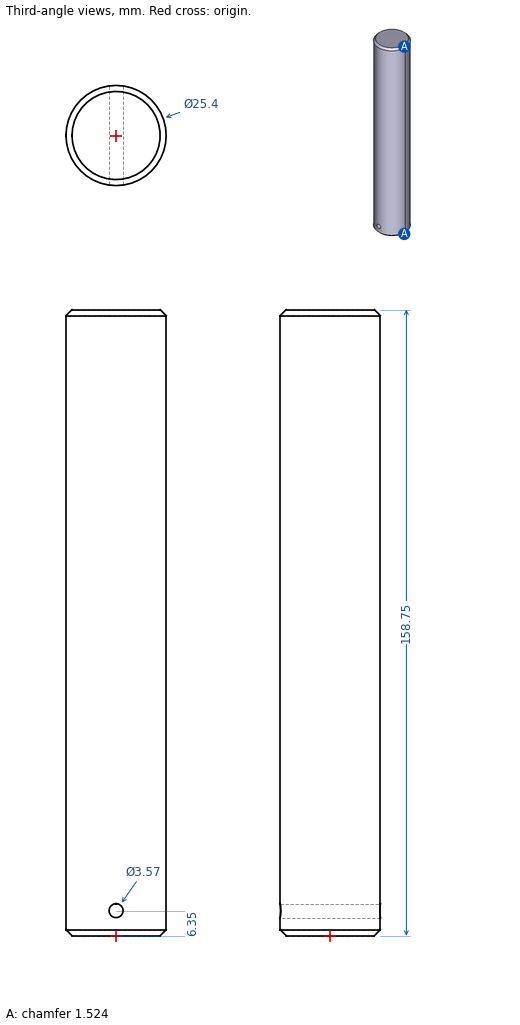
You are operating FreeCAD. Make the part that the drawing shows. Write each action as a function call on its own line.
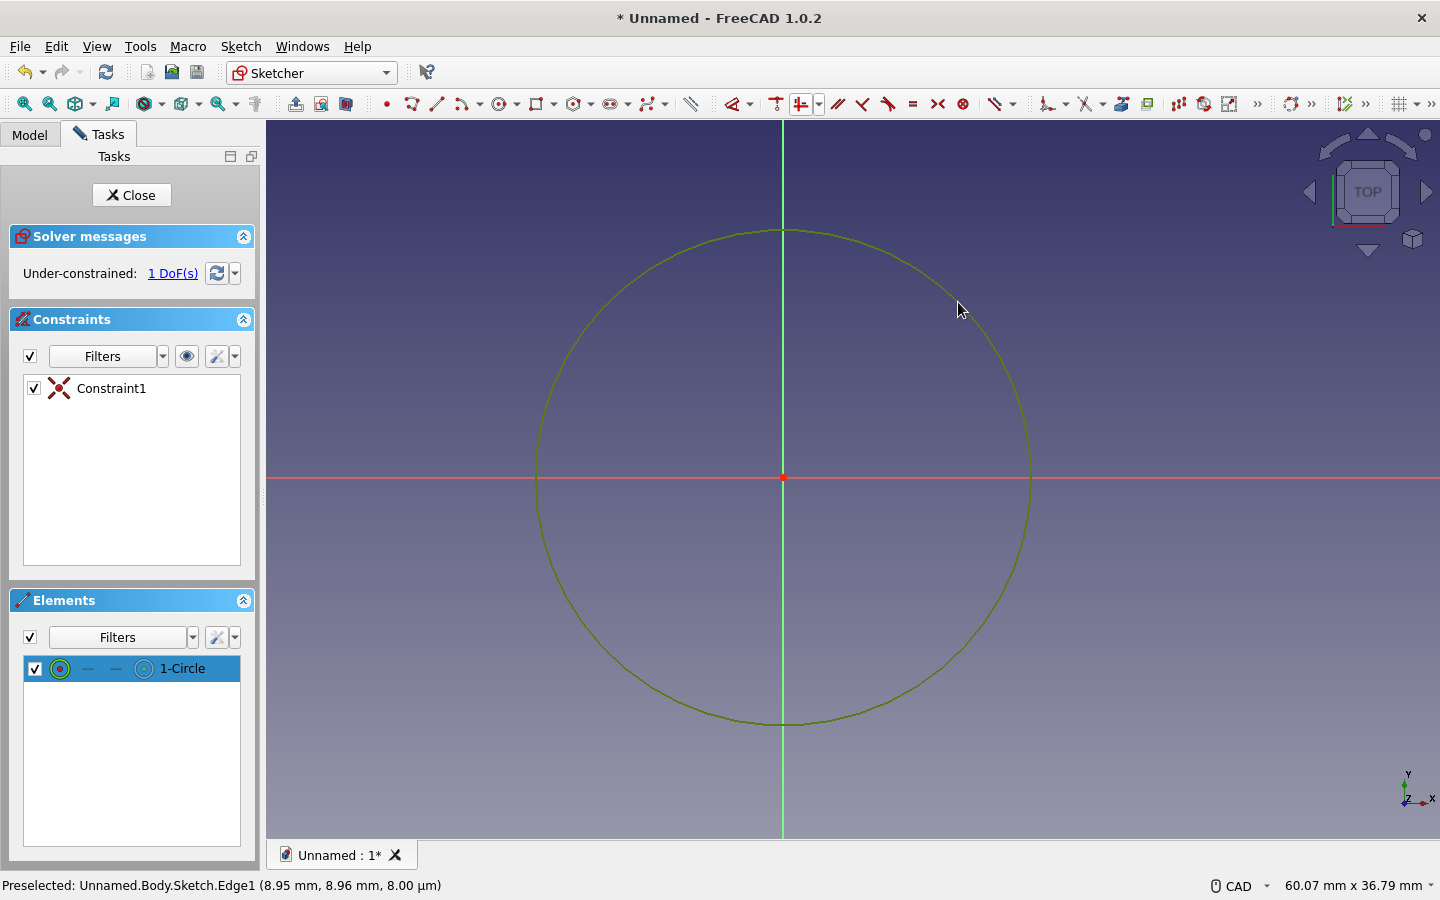
key(k)
key(o)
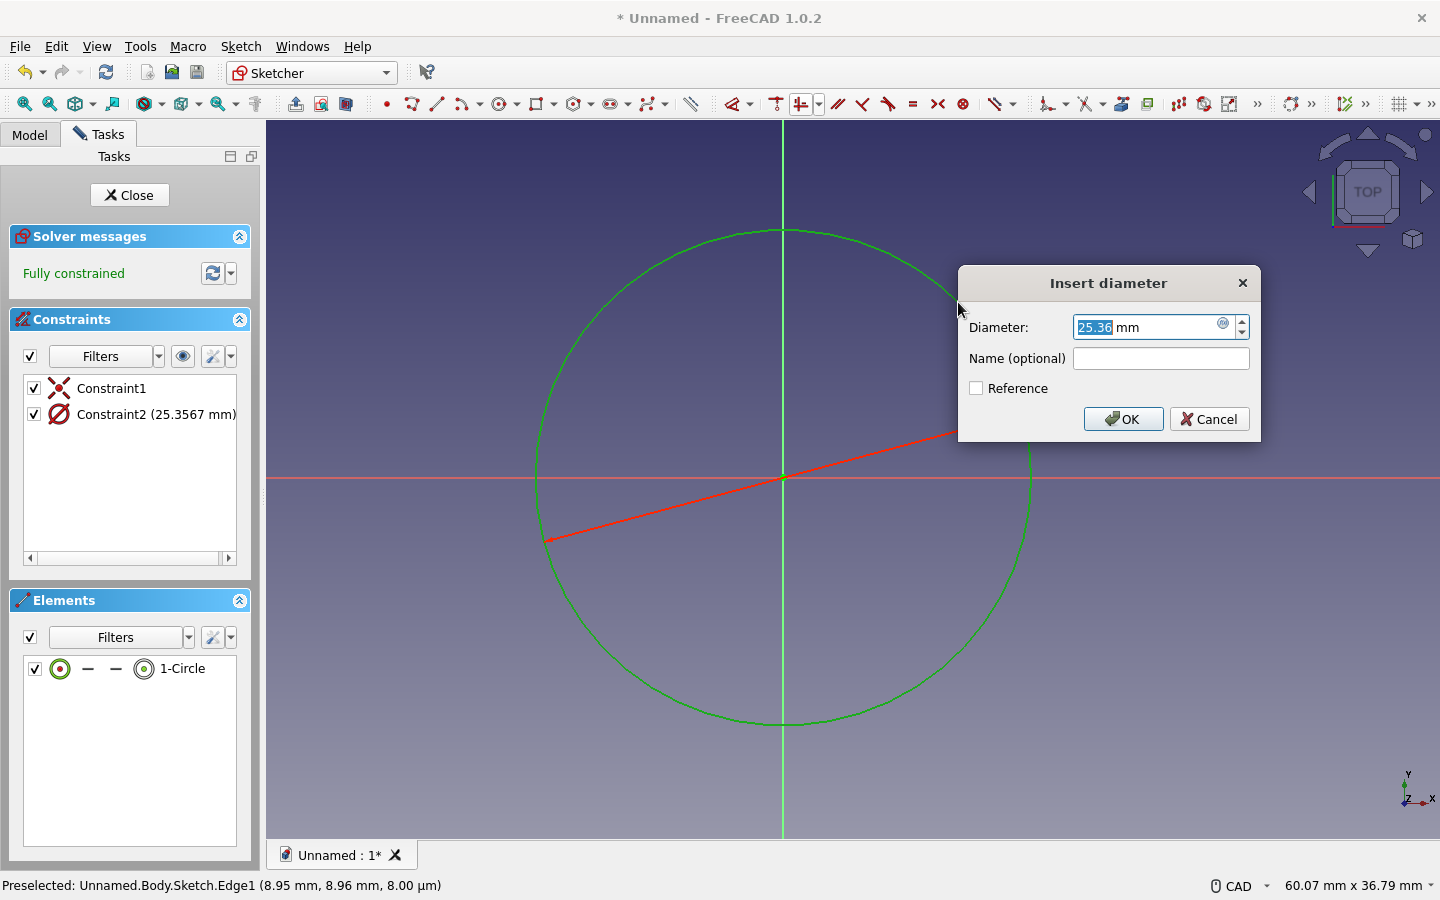
text(25.4)
key(Return)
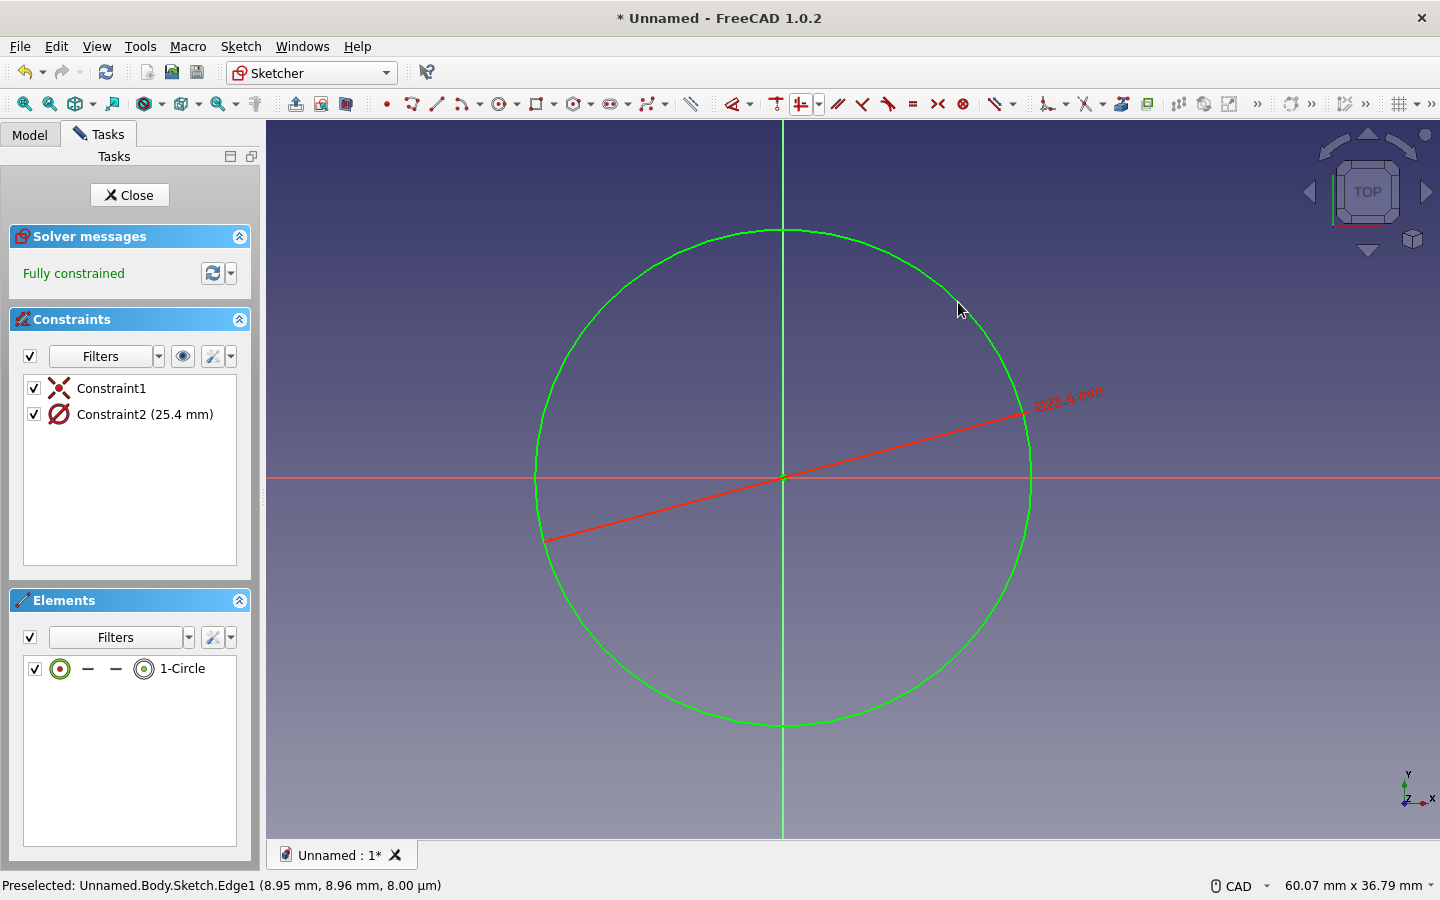
click(130, 195)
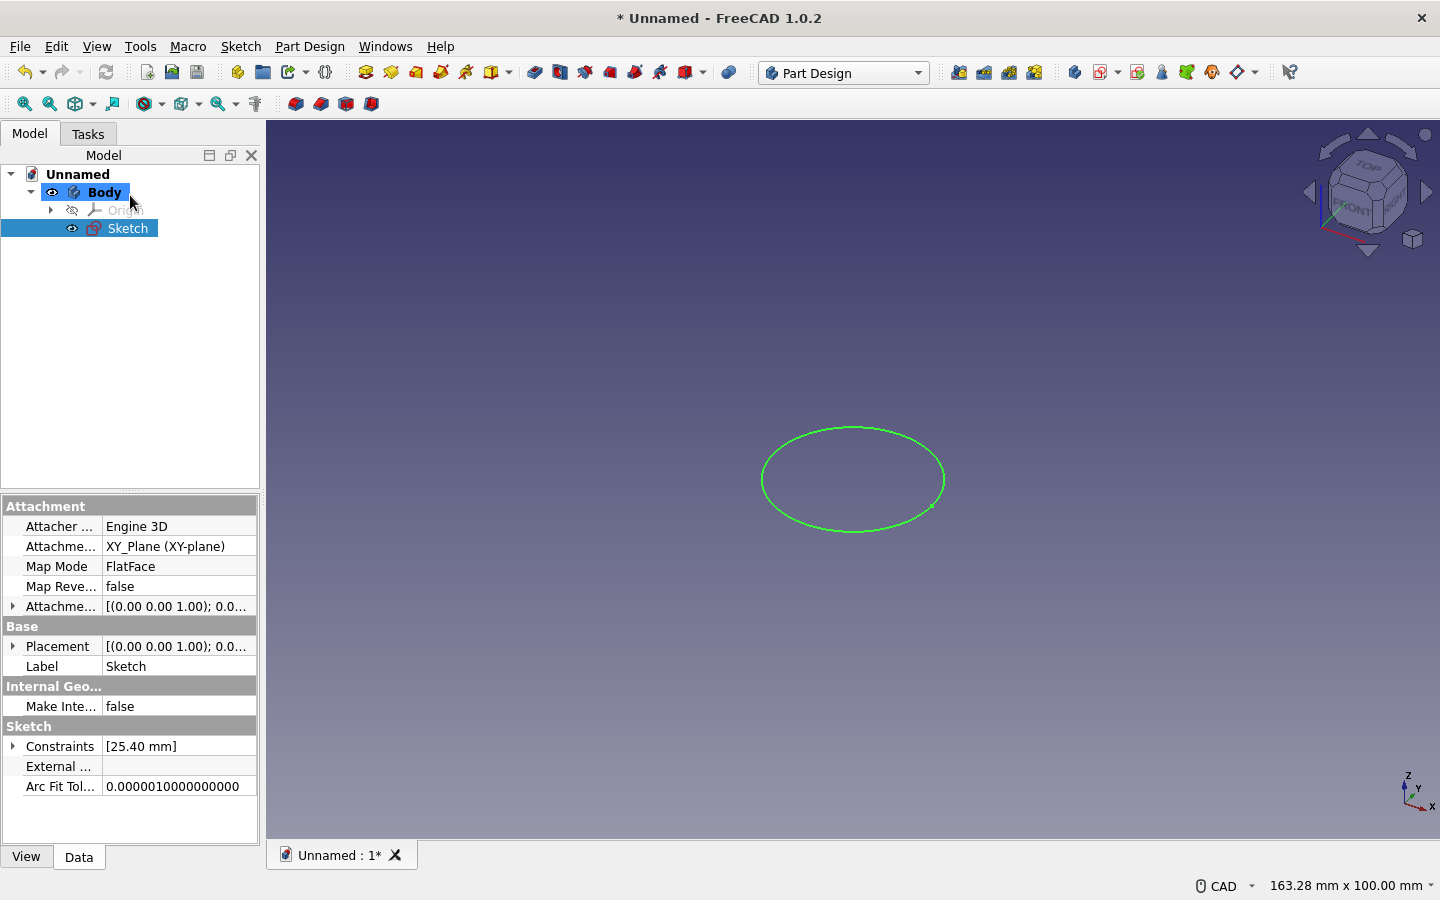
click(366, 72)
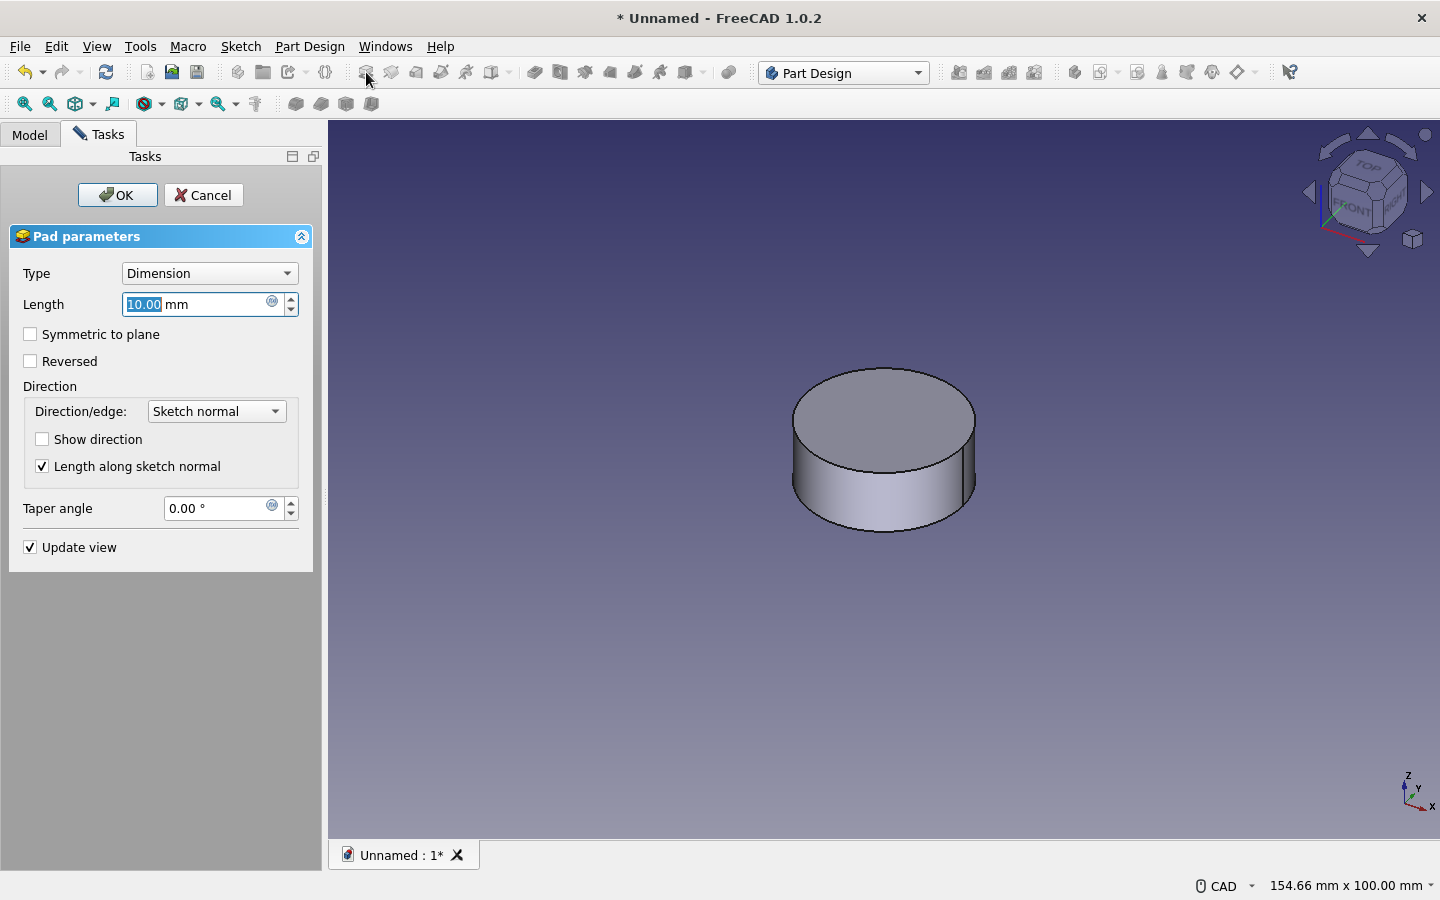
text(158.75)
key(Tab)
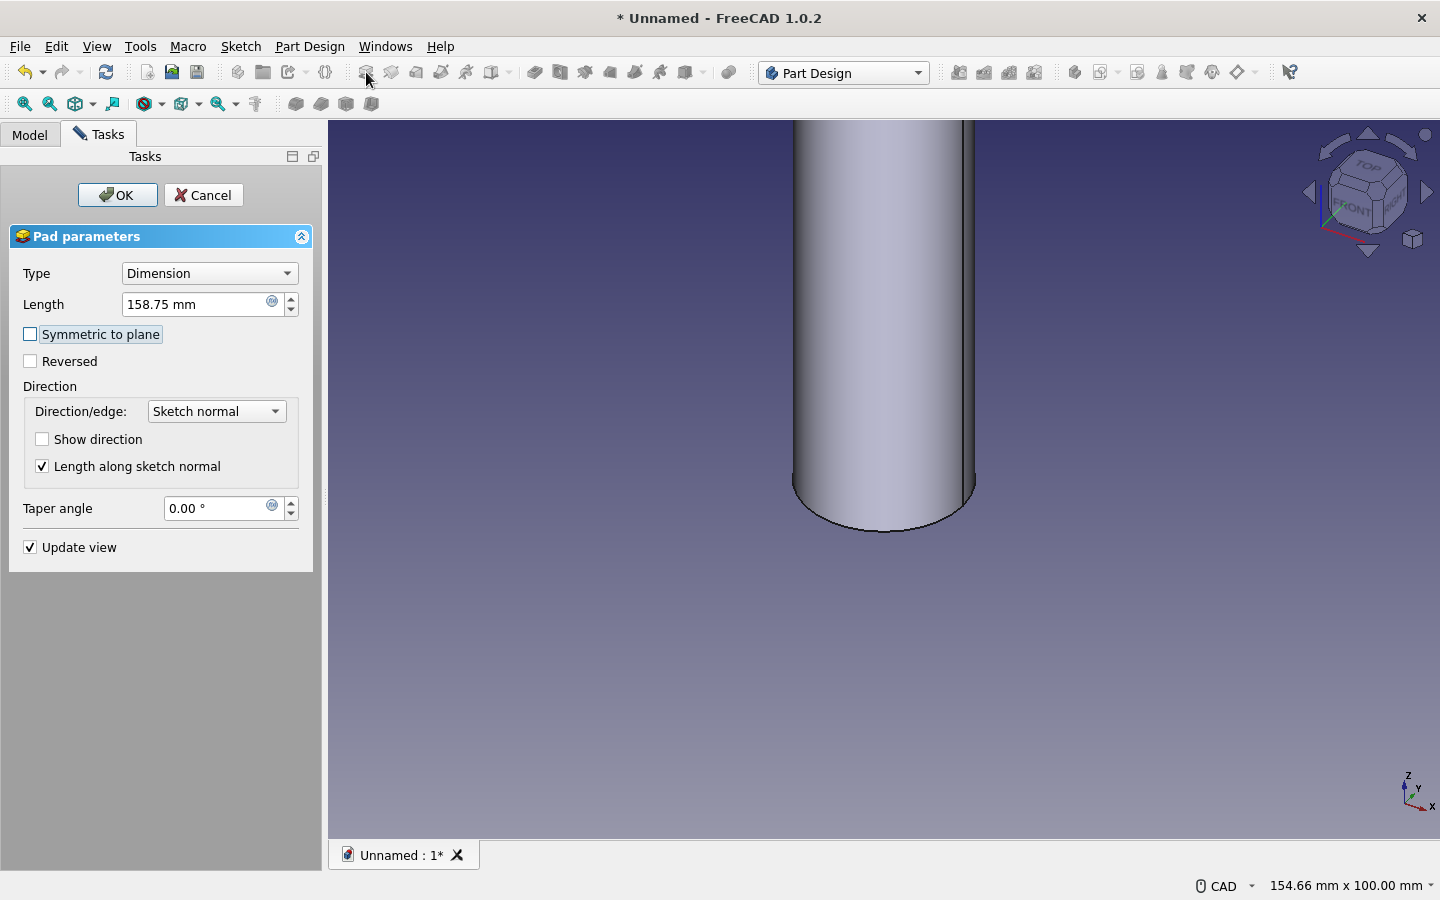
click(118, 195)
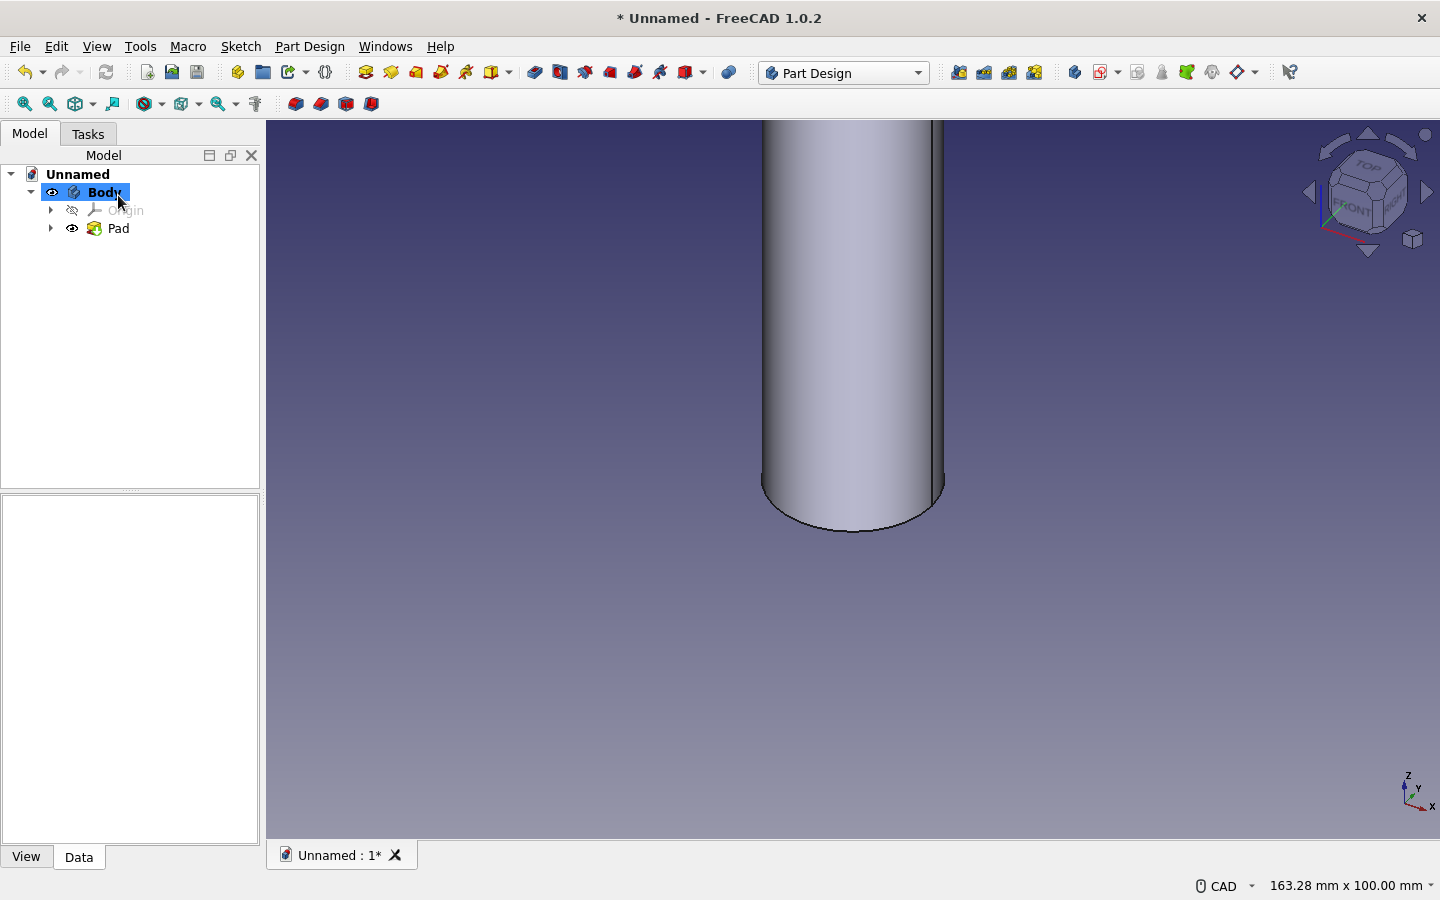
key(v)
key(f)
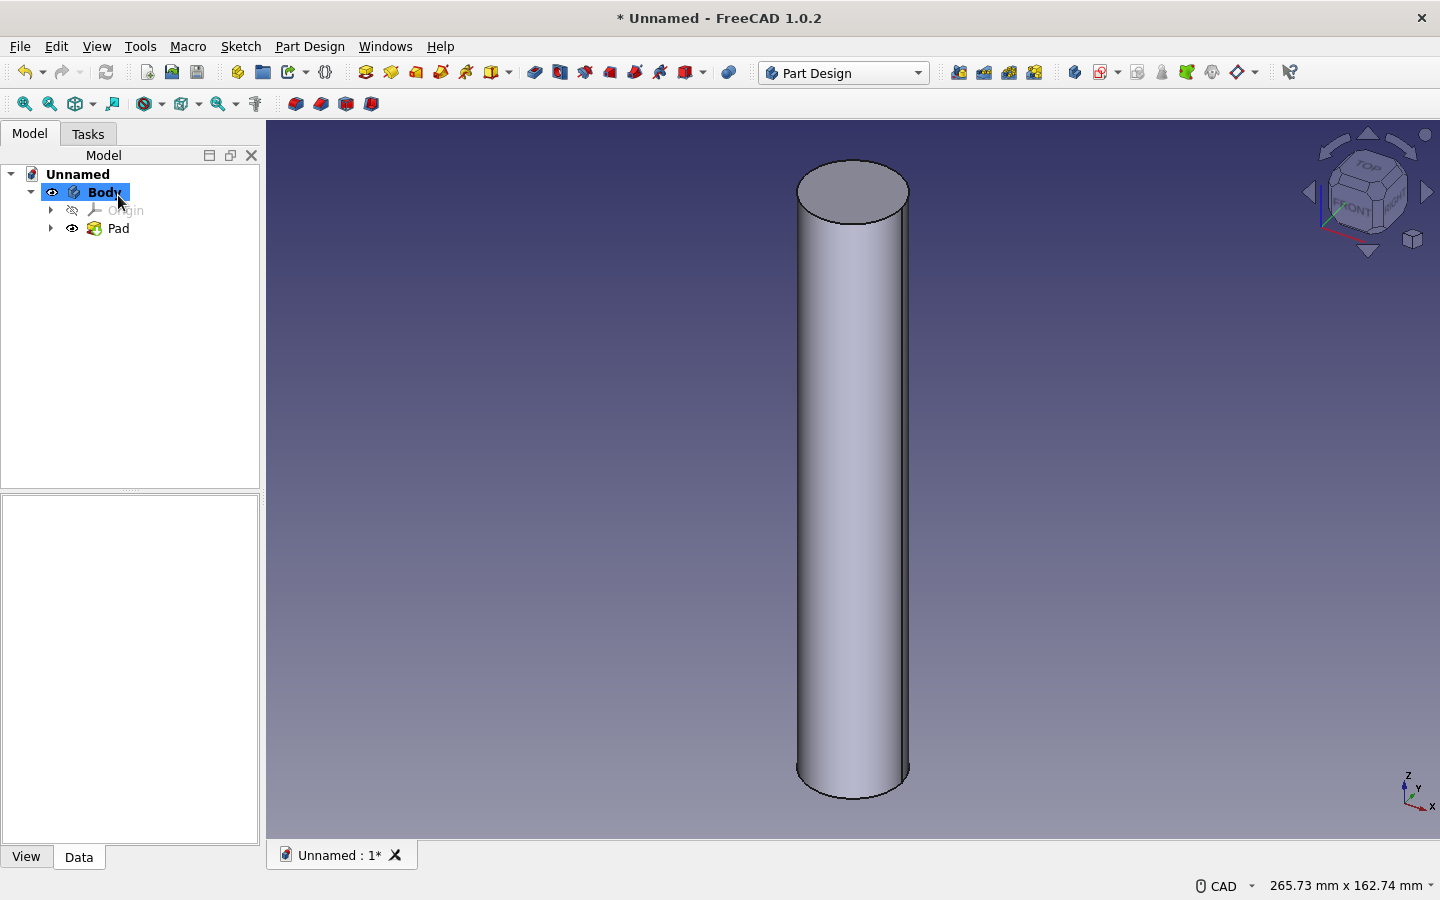
click(797, 195)